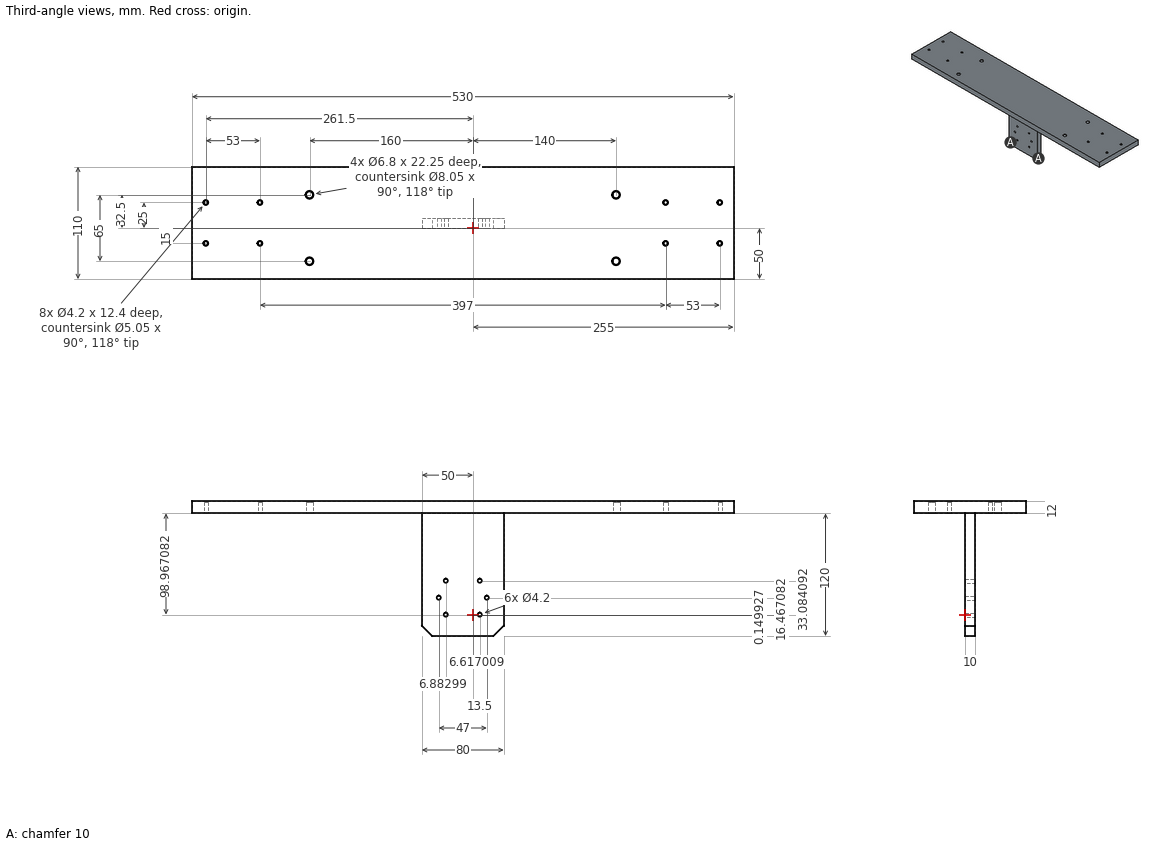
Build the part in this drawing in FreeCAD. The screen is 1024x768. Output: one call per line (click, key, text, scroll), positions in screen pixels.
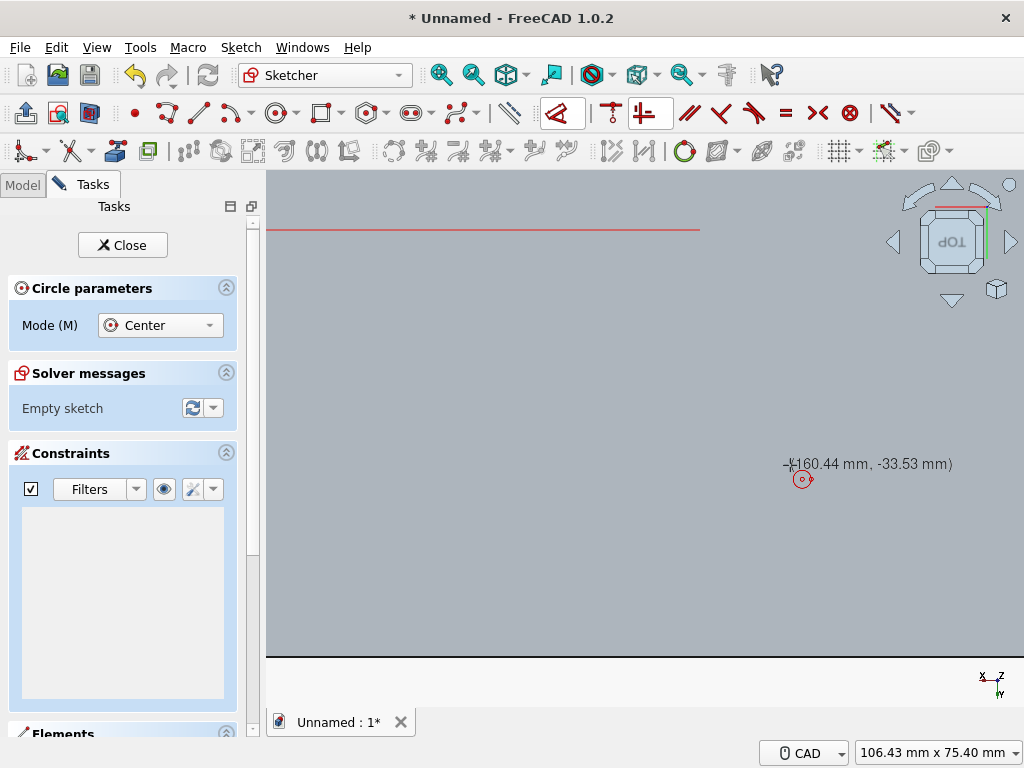
scroll(747, 480, down, 9)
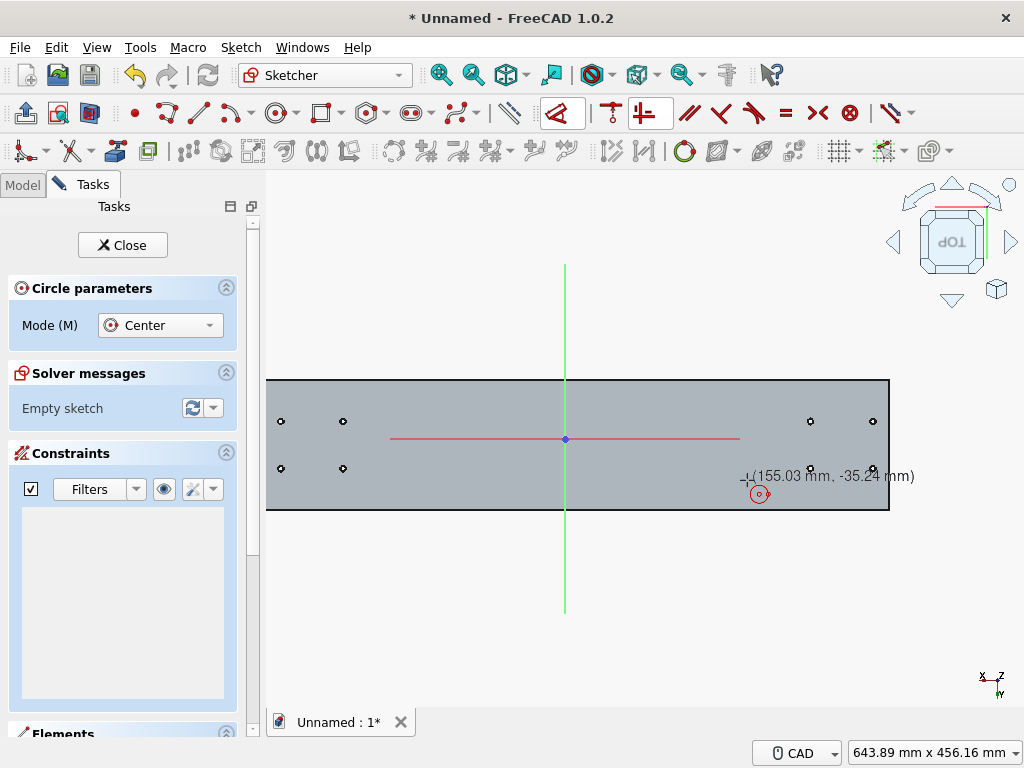
click(753, 477)
move(756, 475)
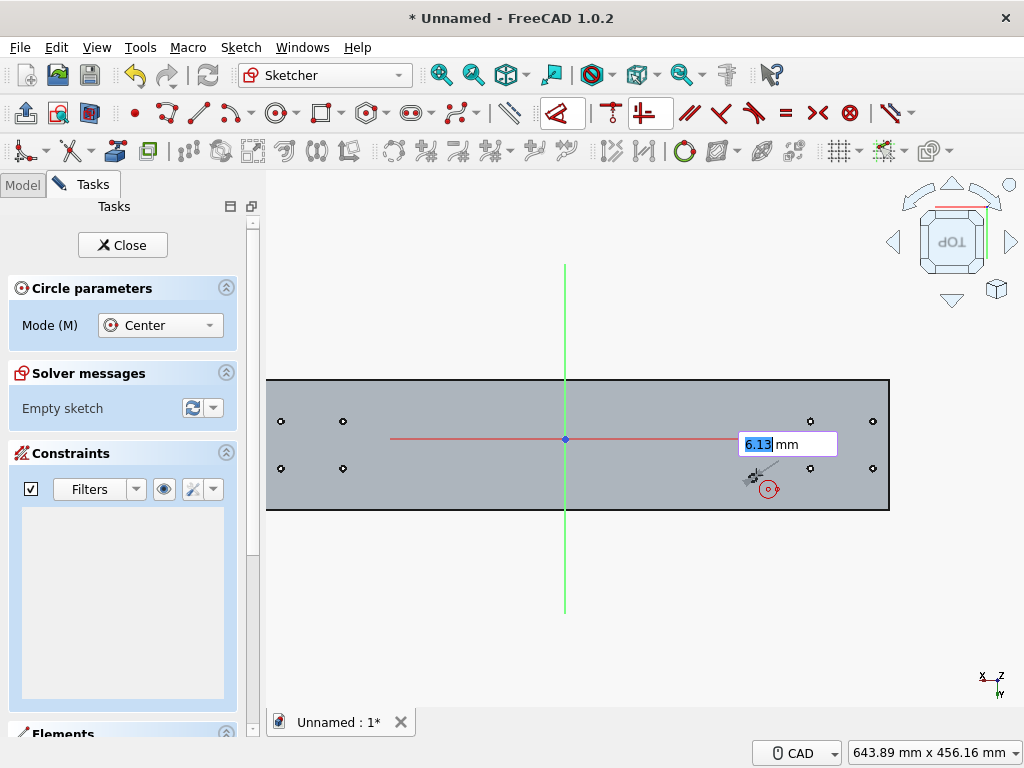
text(6.8)
key(Return)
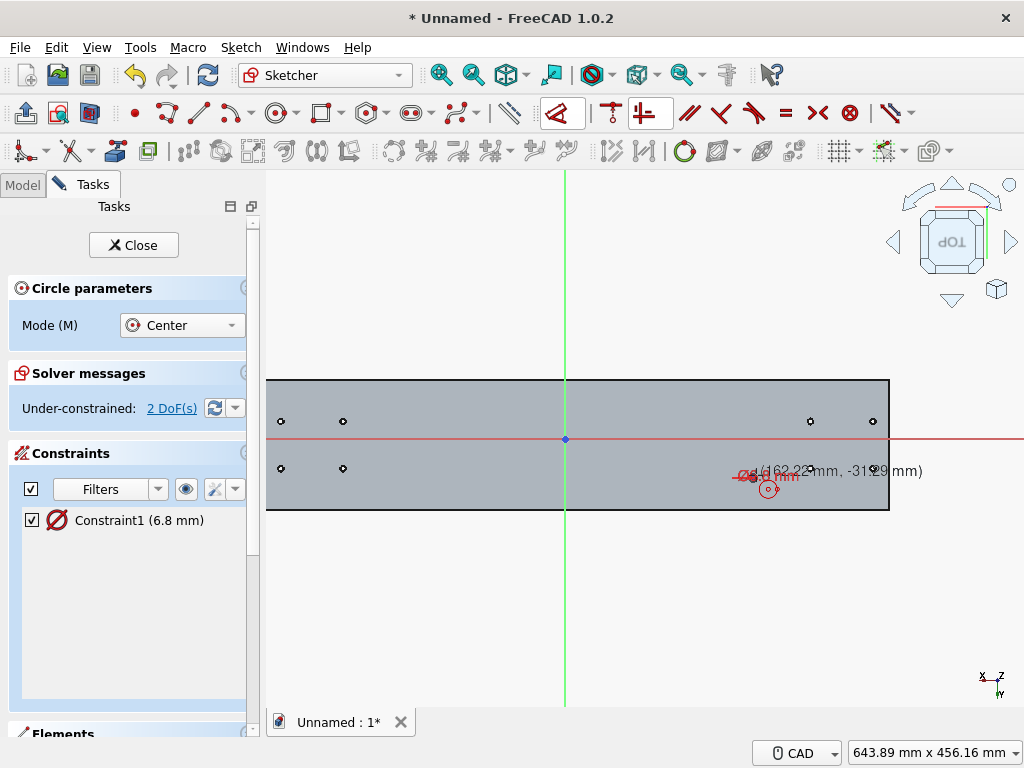
scroll(753, 401, up, 9)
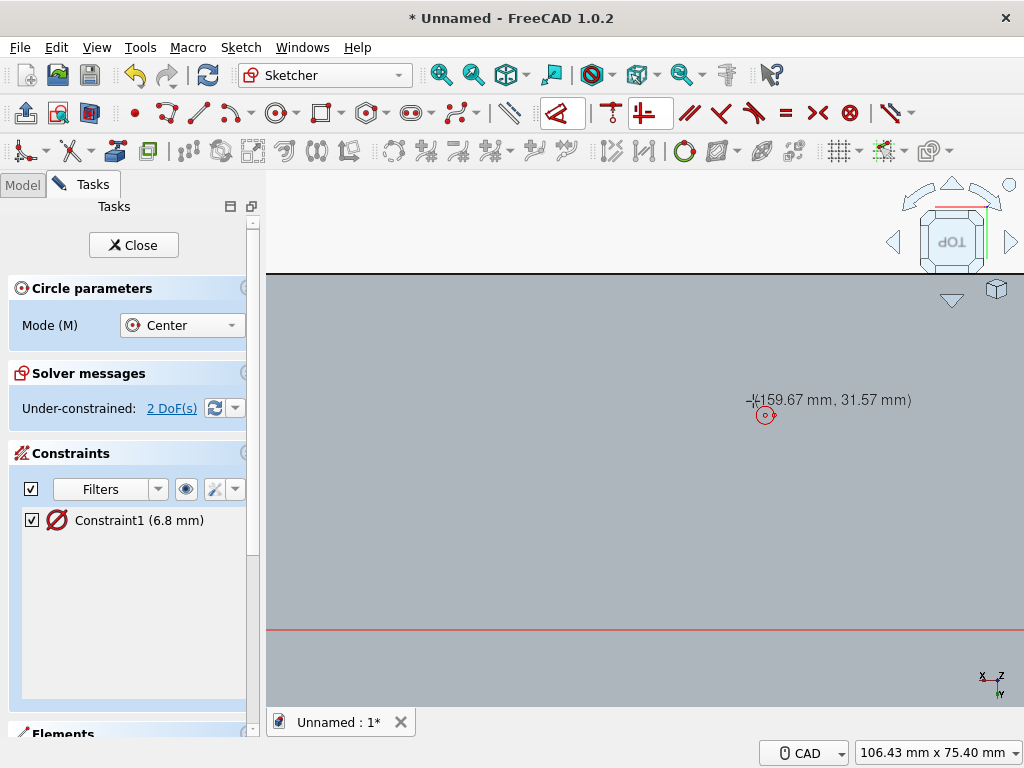
scroll(753, 401, down, 9)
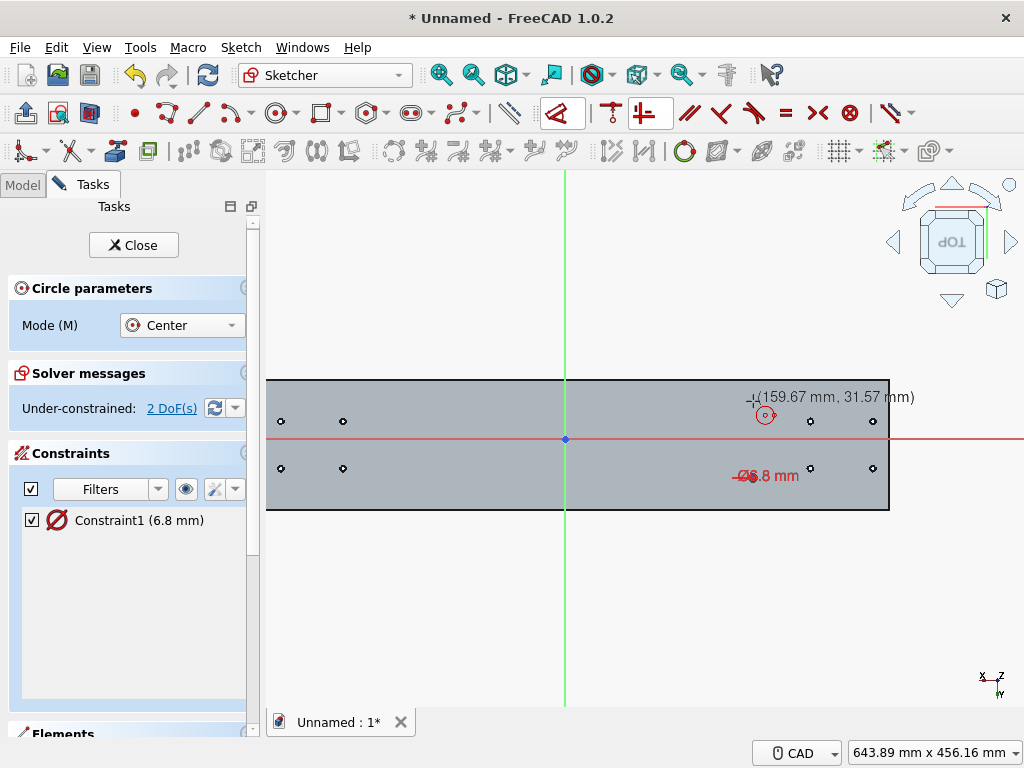
click(753, 401)
move(756, 398)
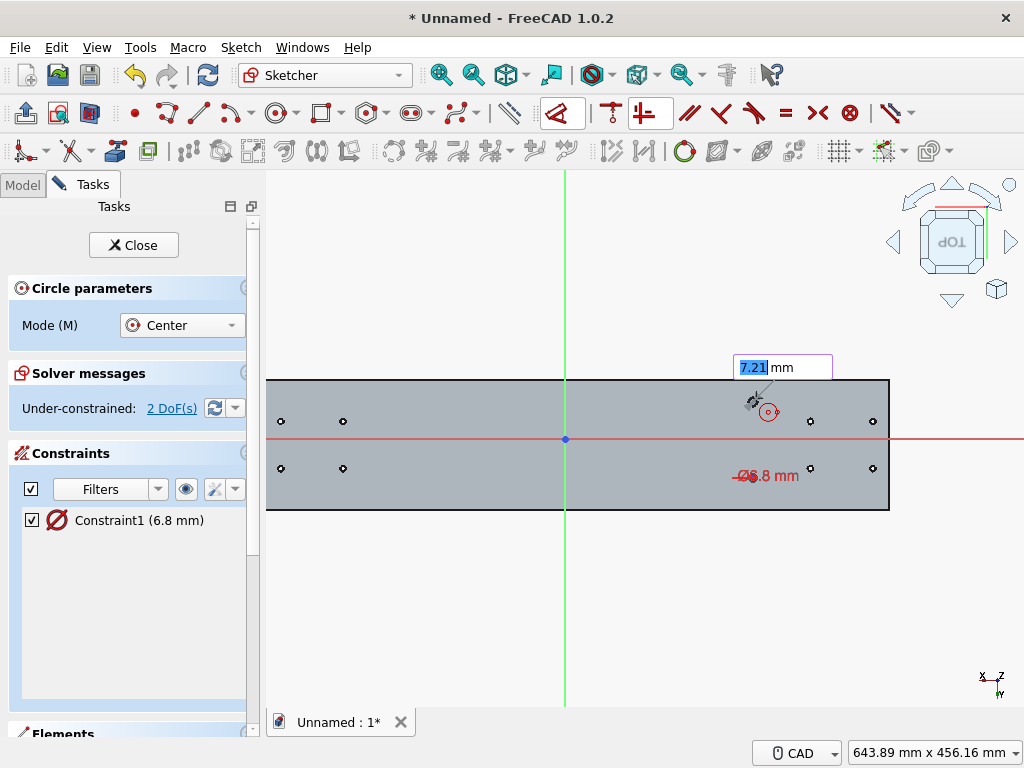
text(6.8)
key(Return)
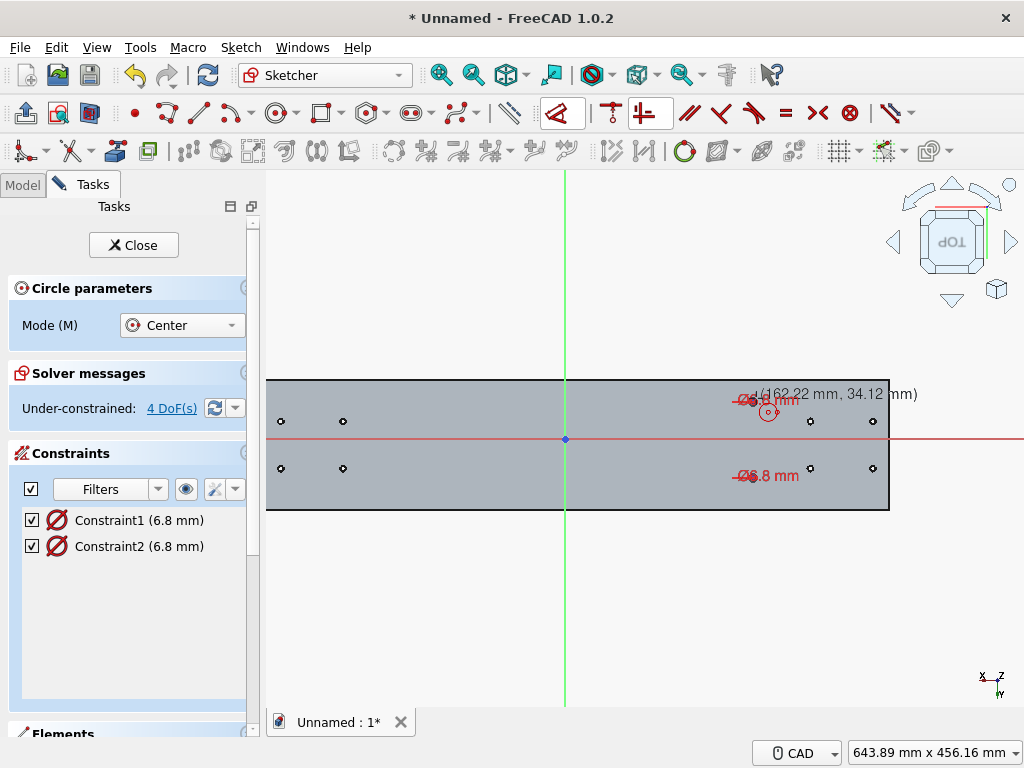
scroll(400, 477, up, 9)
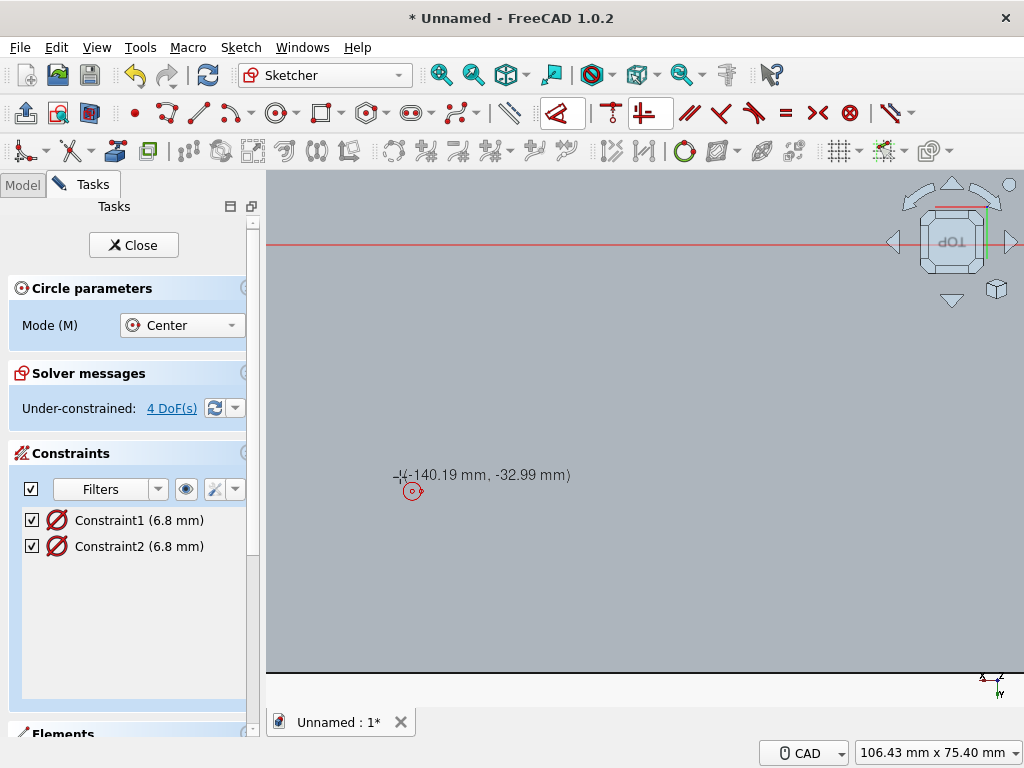
scroll(400, 477, down, 9)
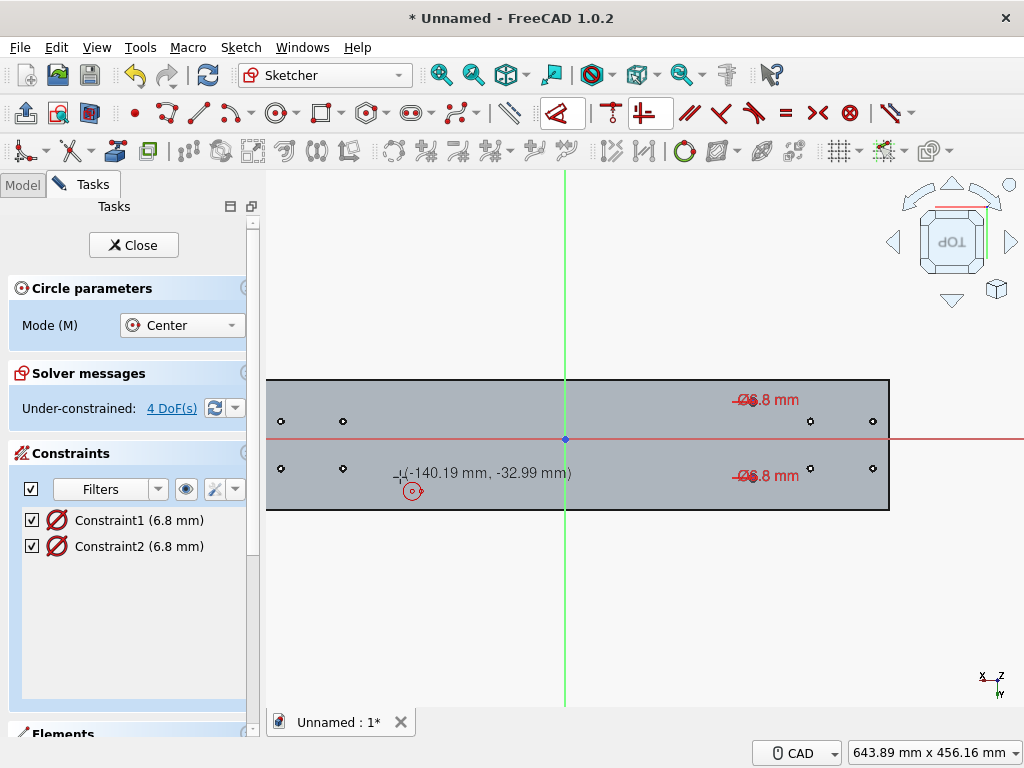
click(400, 477)
move(403, 475)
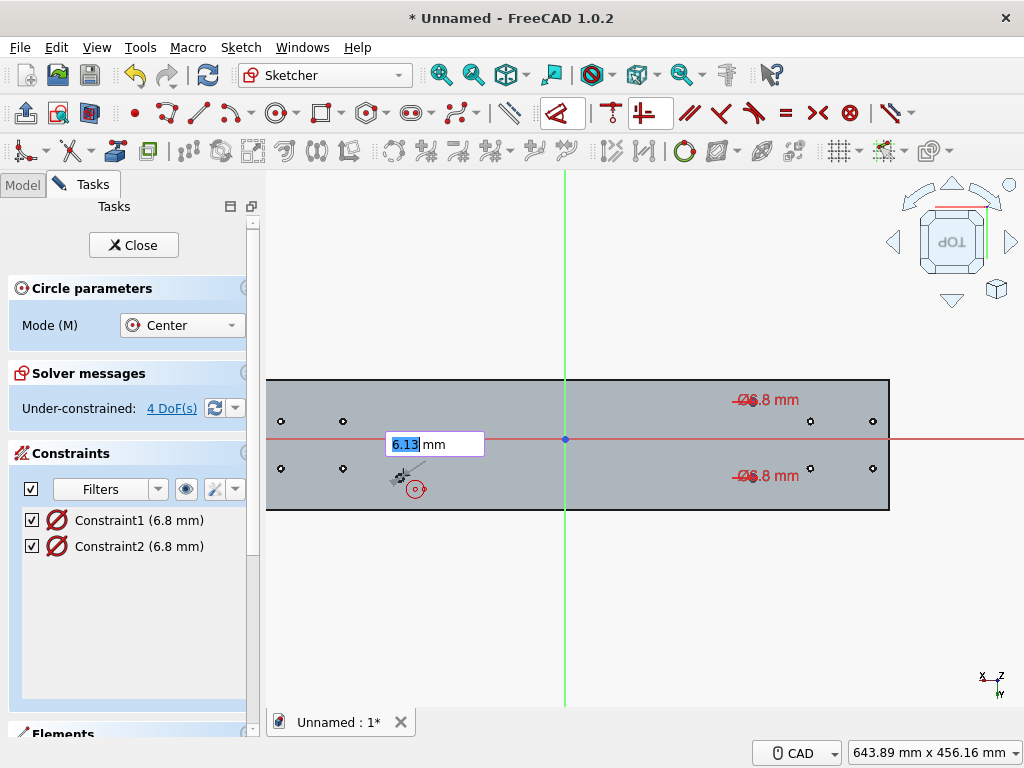
text(6.8)
key(Return)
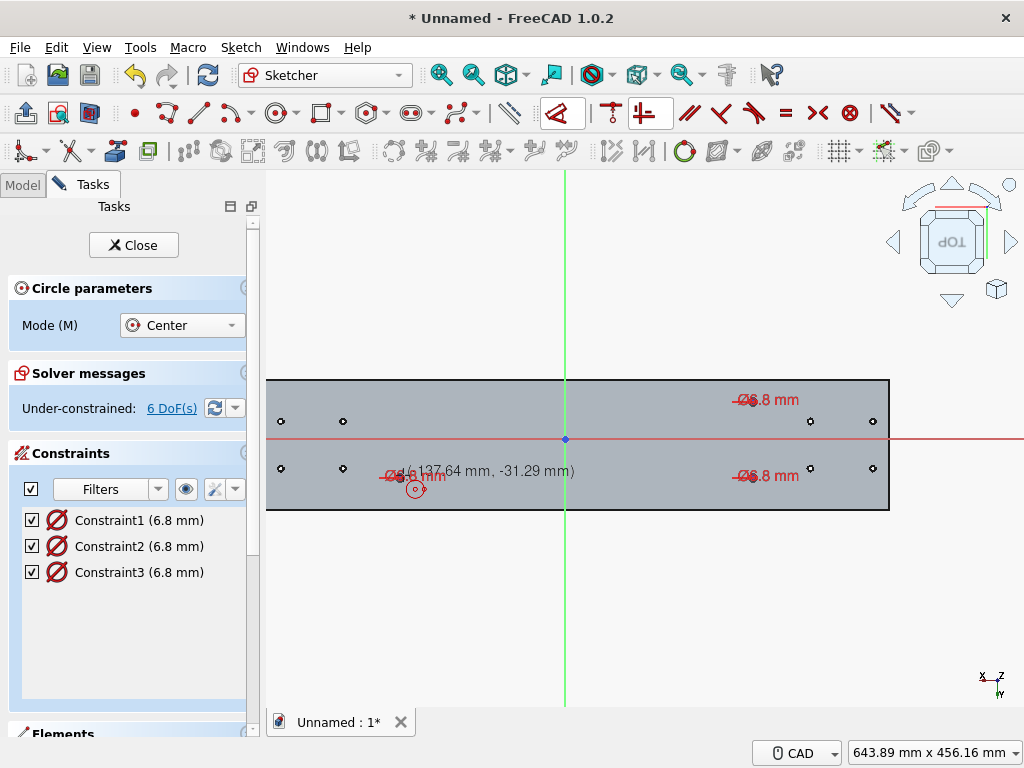
scroll(400, 401, up, 9)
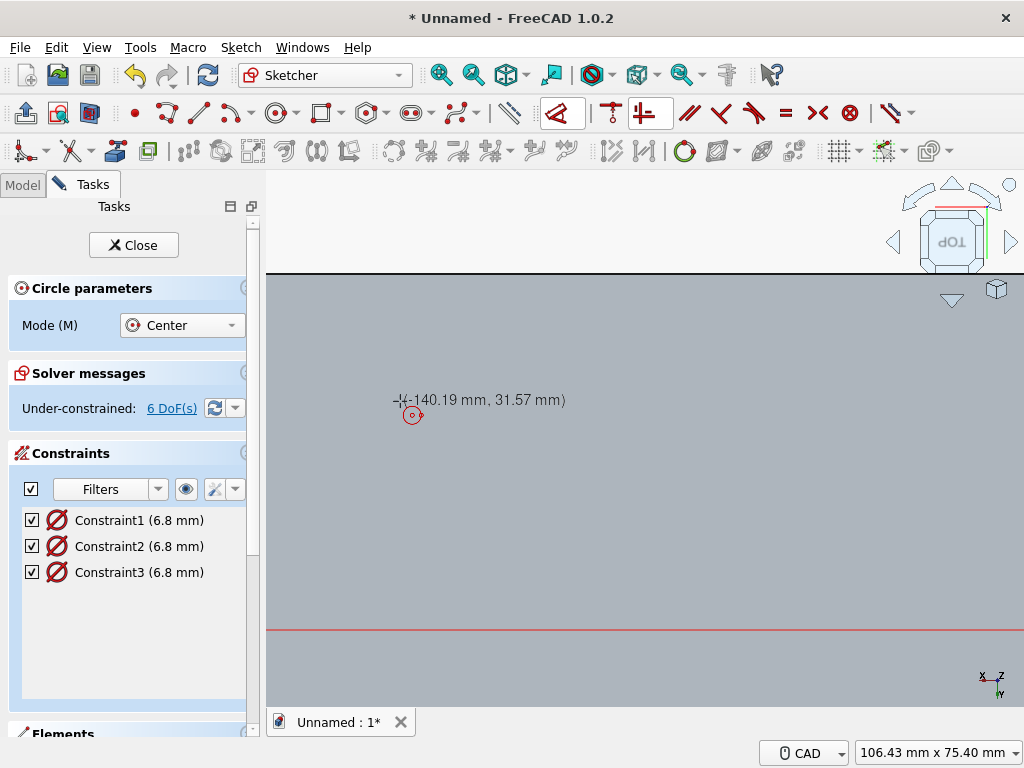
scroll(400, 401, down, 9)